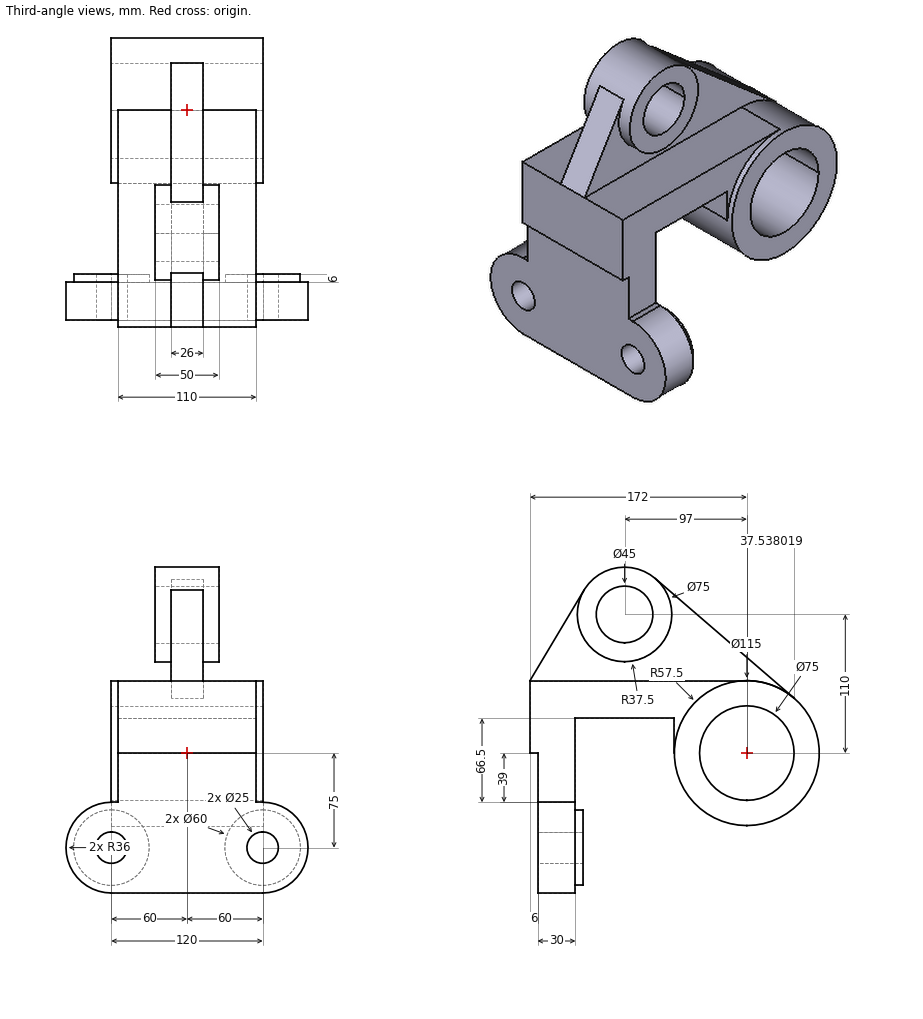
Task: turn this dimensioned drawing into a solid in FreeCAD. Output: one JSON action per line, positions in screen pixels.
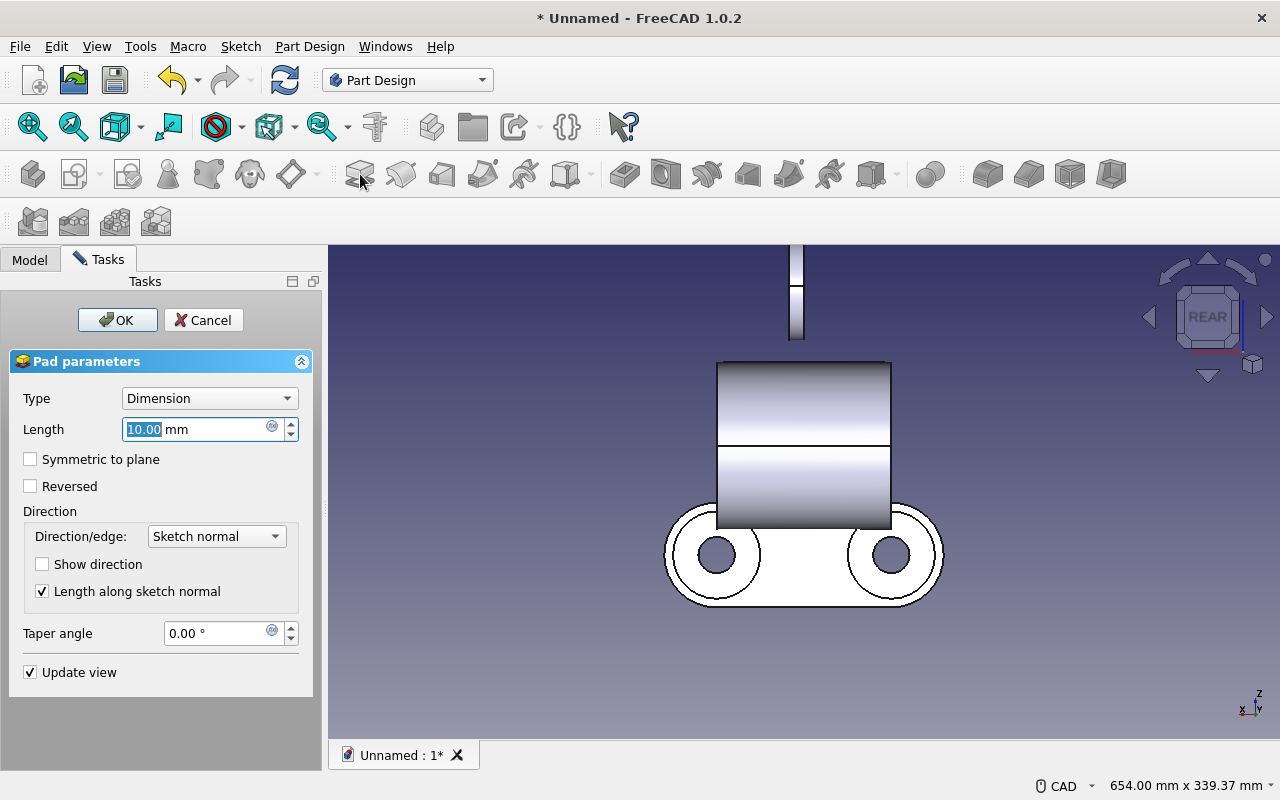
{"action": "type", "text": "50"}
{"action": "key", "text": "Tab"}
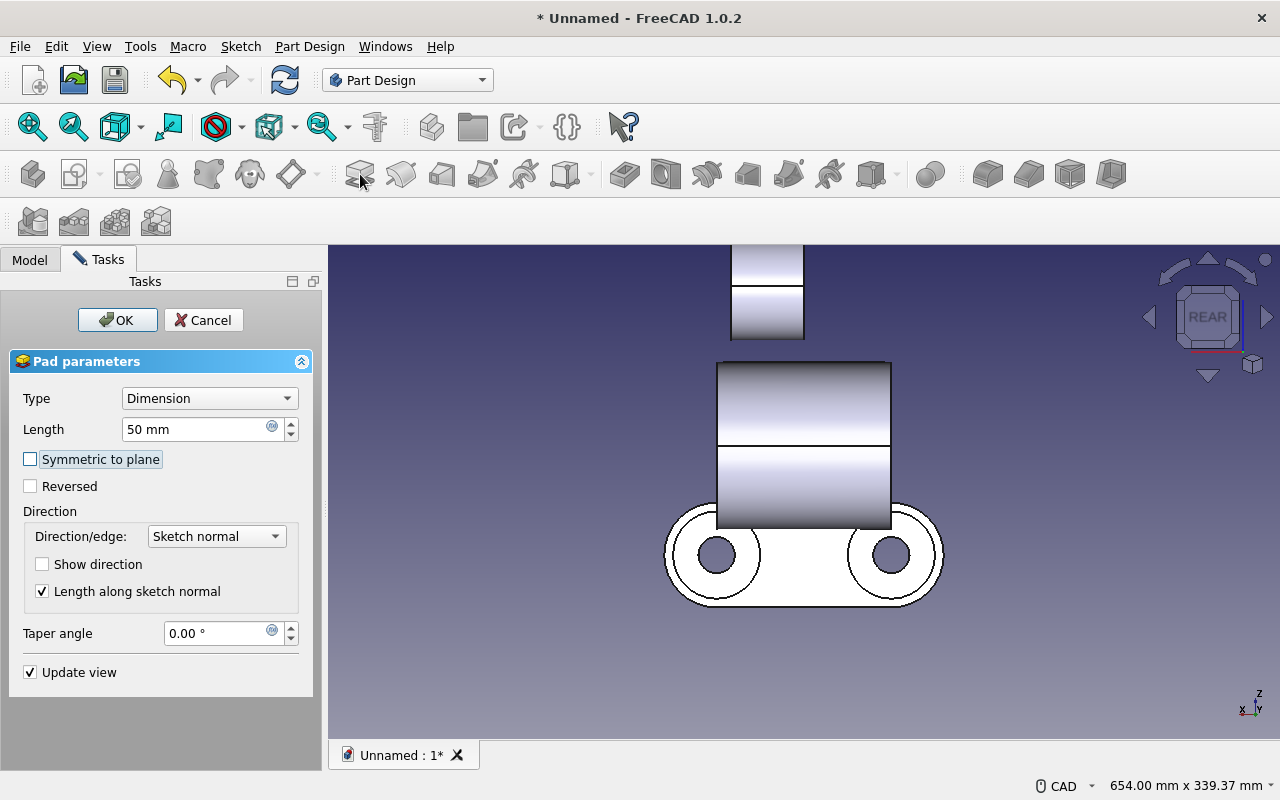
{"action": "left_click", "coordinate": [31, 459]}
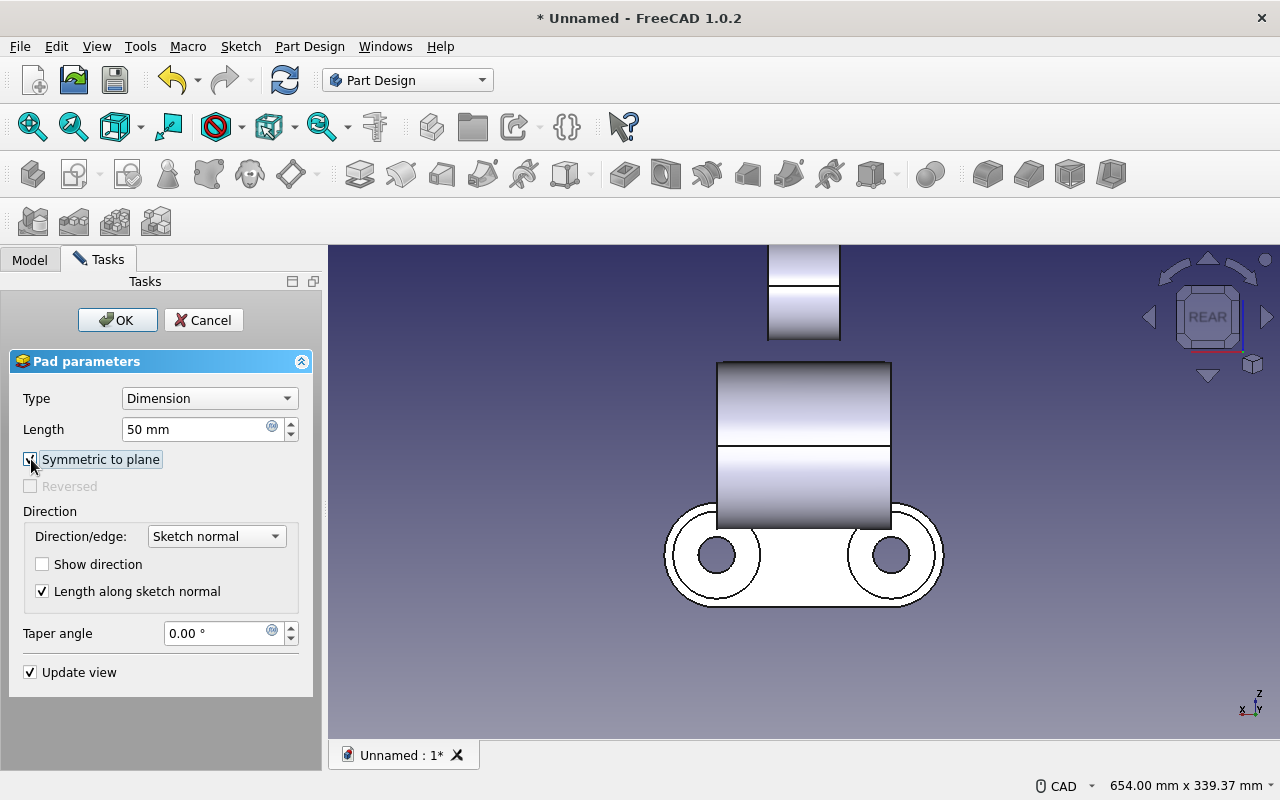
{"action": "left_click", "coordinate": [118, 320]}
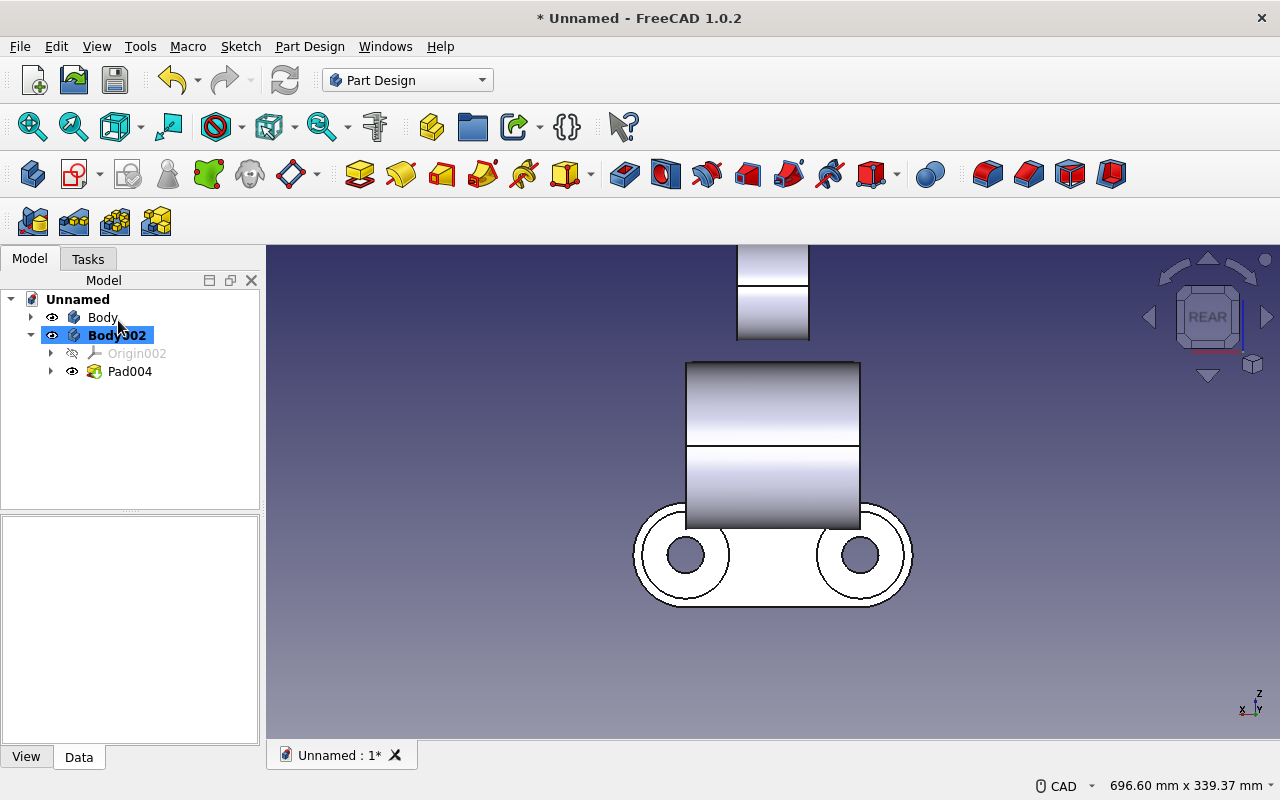
{"action": "left_click", "coordinate": [33, 128]}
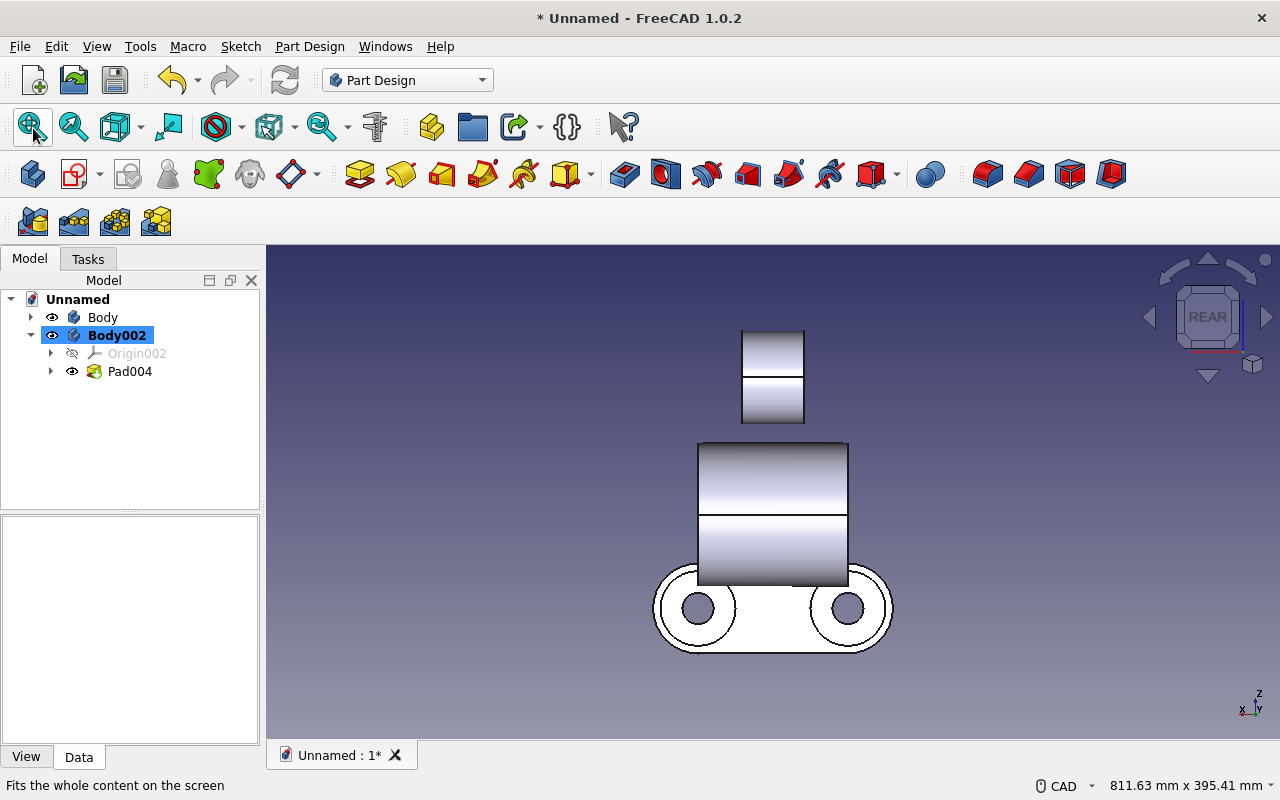
{"action": "double_click", "coordinate": [97, 317]}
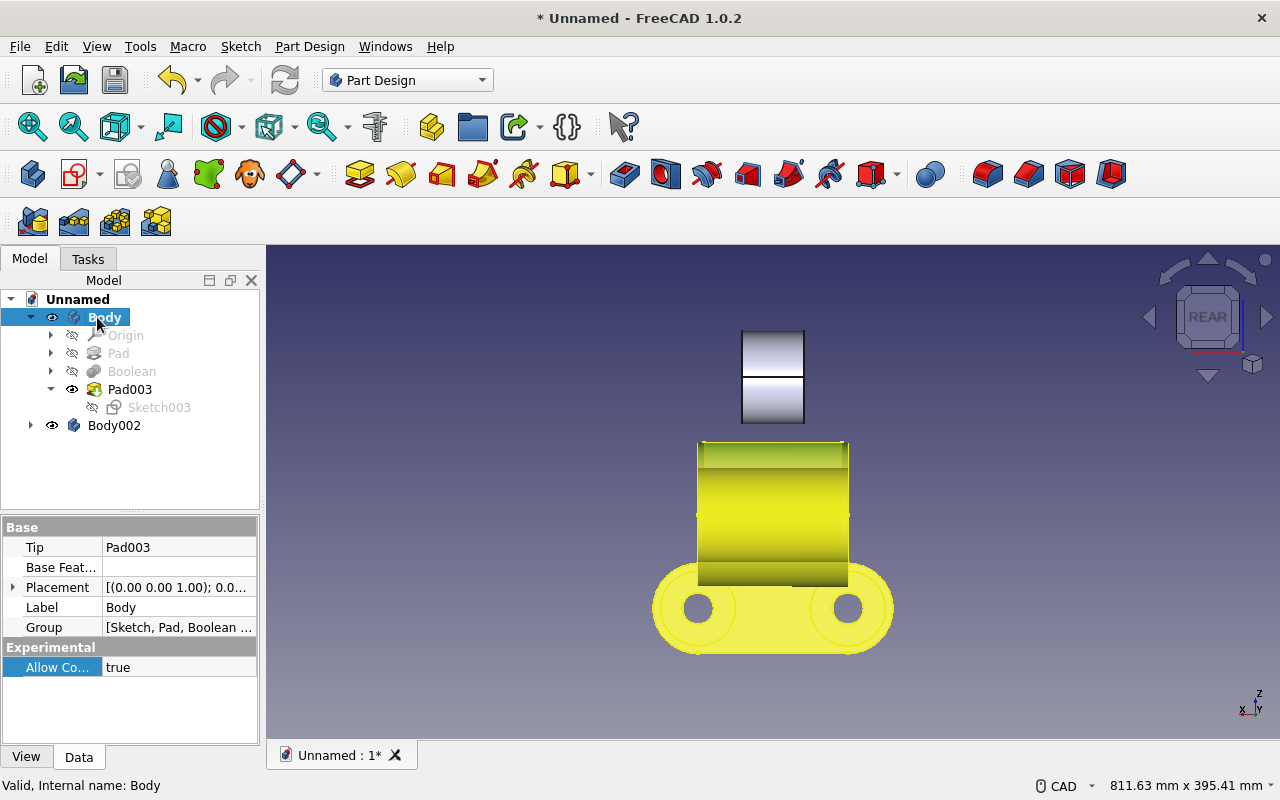
{"action": "left_click", "coordinate": [97, 425]}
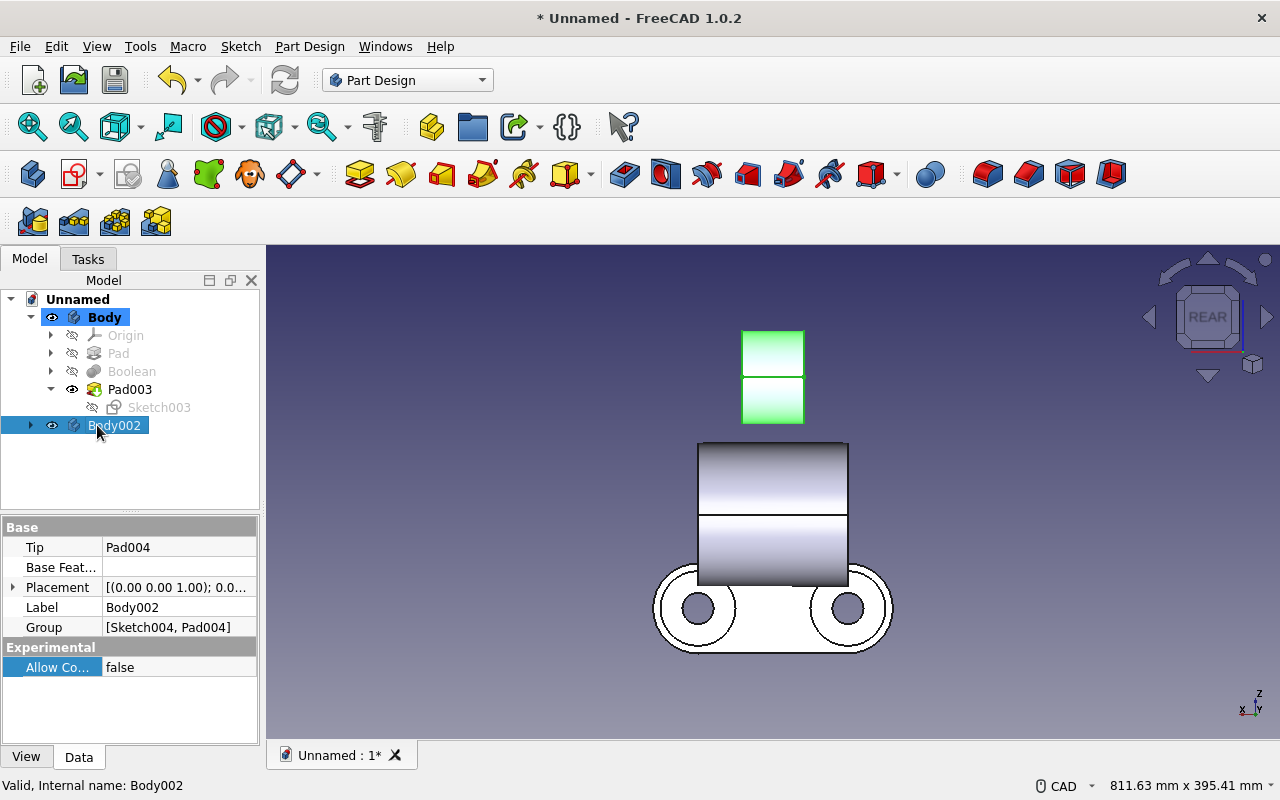
{"action": "left_click", "coordinate": [931, 174]}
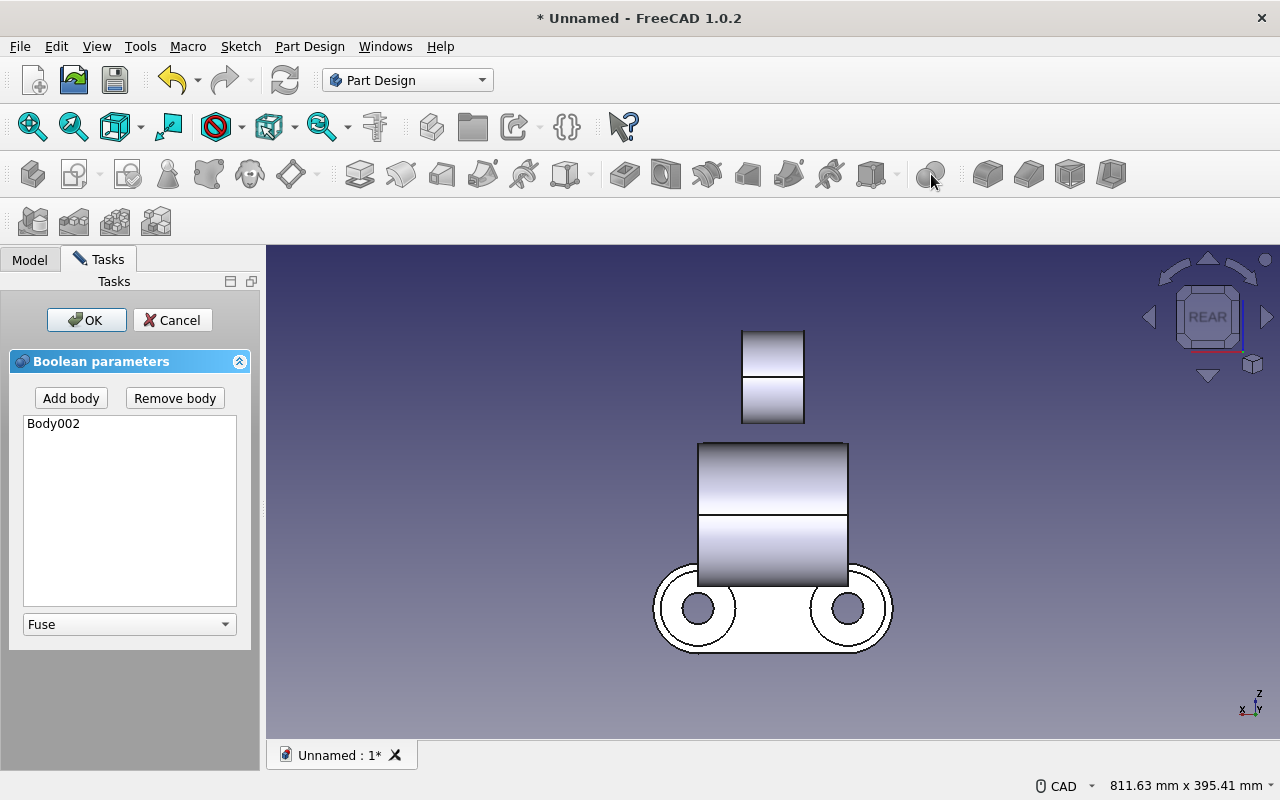
{"action": "left_click", "coordinate": [87, 320]}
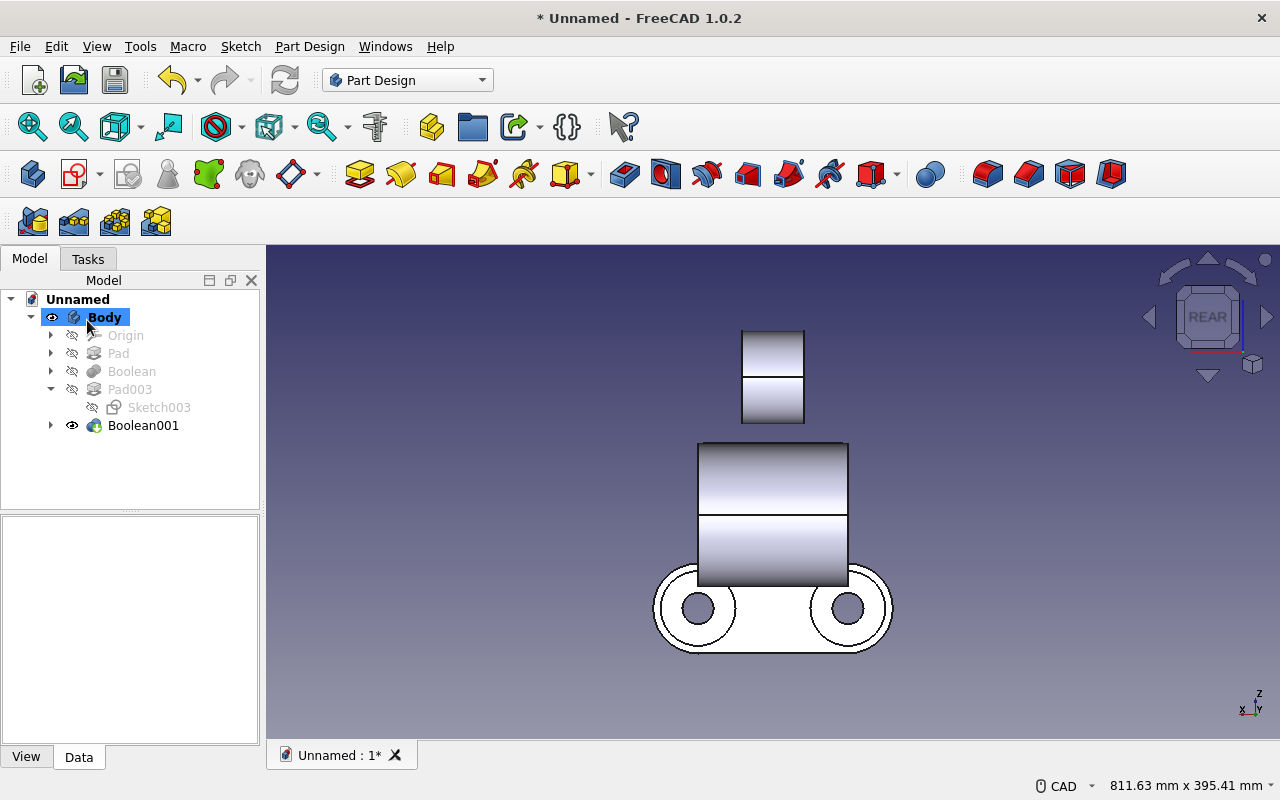
{"action": "left_click", "coordinate": [74, 174]}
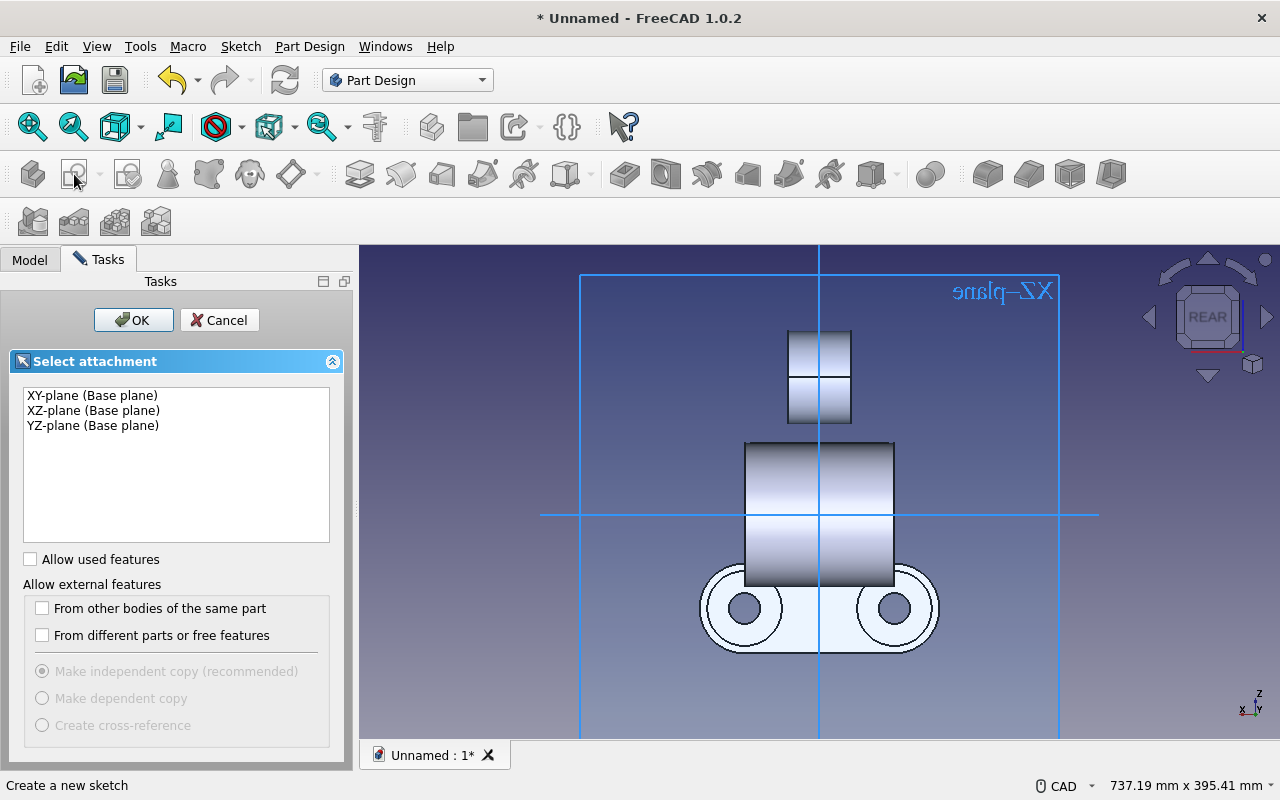
{"action": "left_click", "coordinate": [84, 426]}